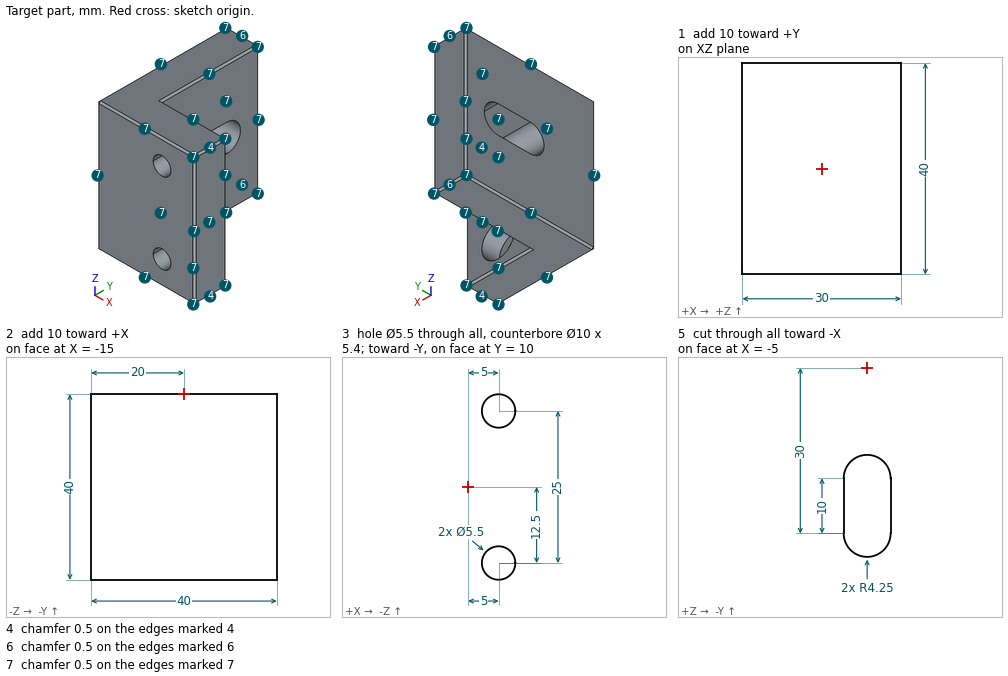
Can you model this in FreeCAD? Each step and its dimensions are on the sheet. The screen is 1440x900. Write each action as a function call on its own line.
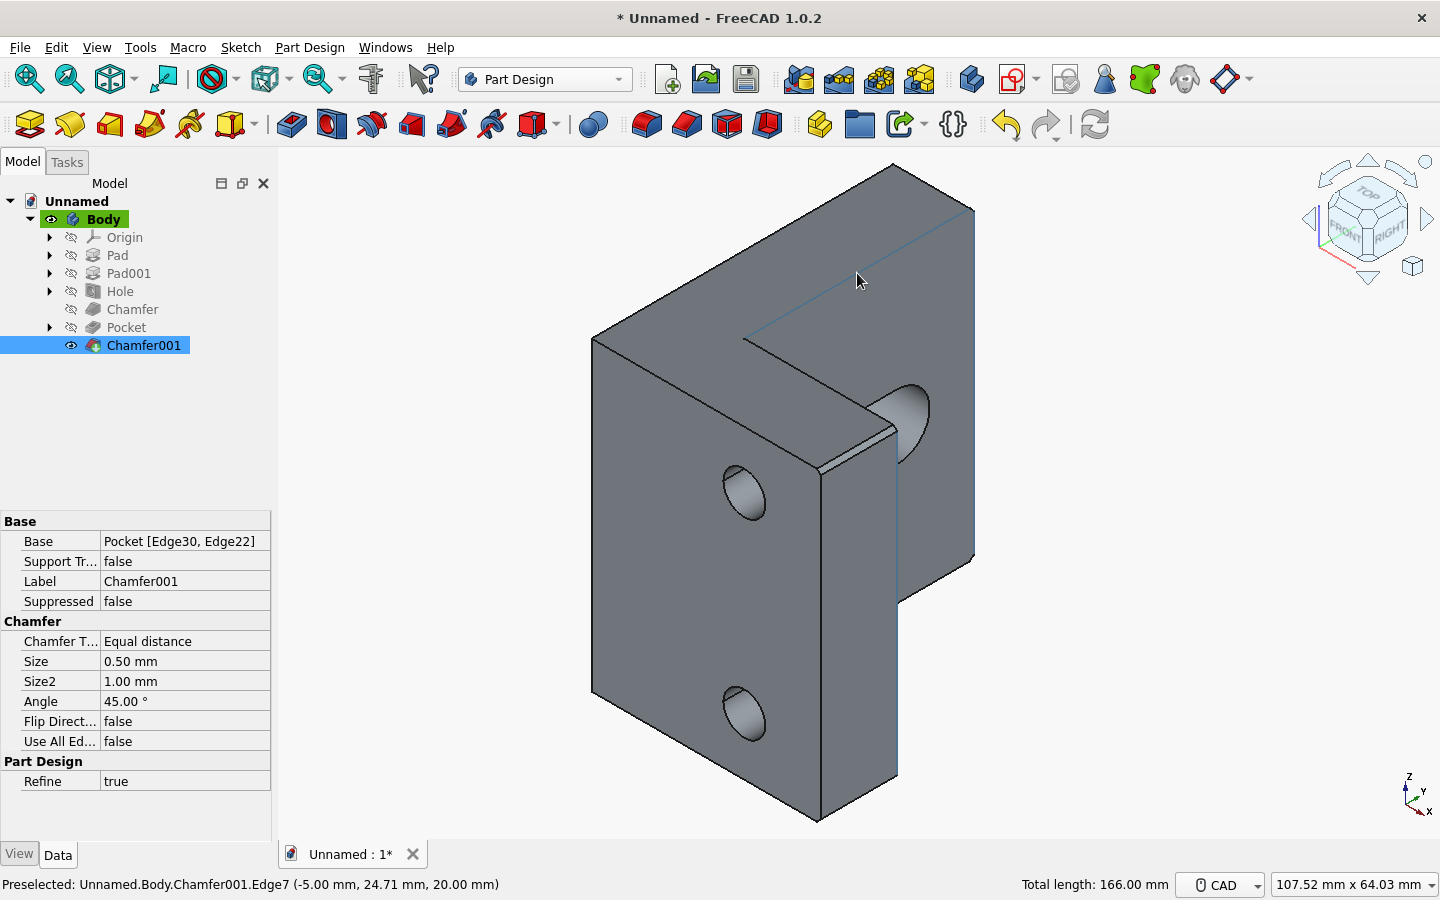
click(704, 403, ctrl)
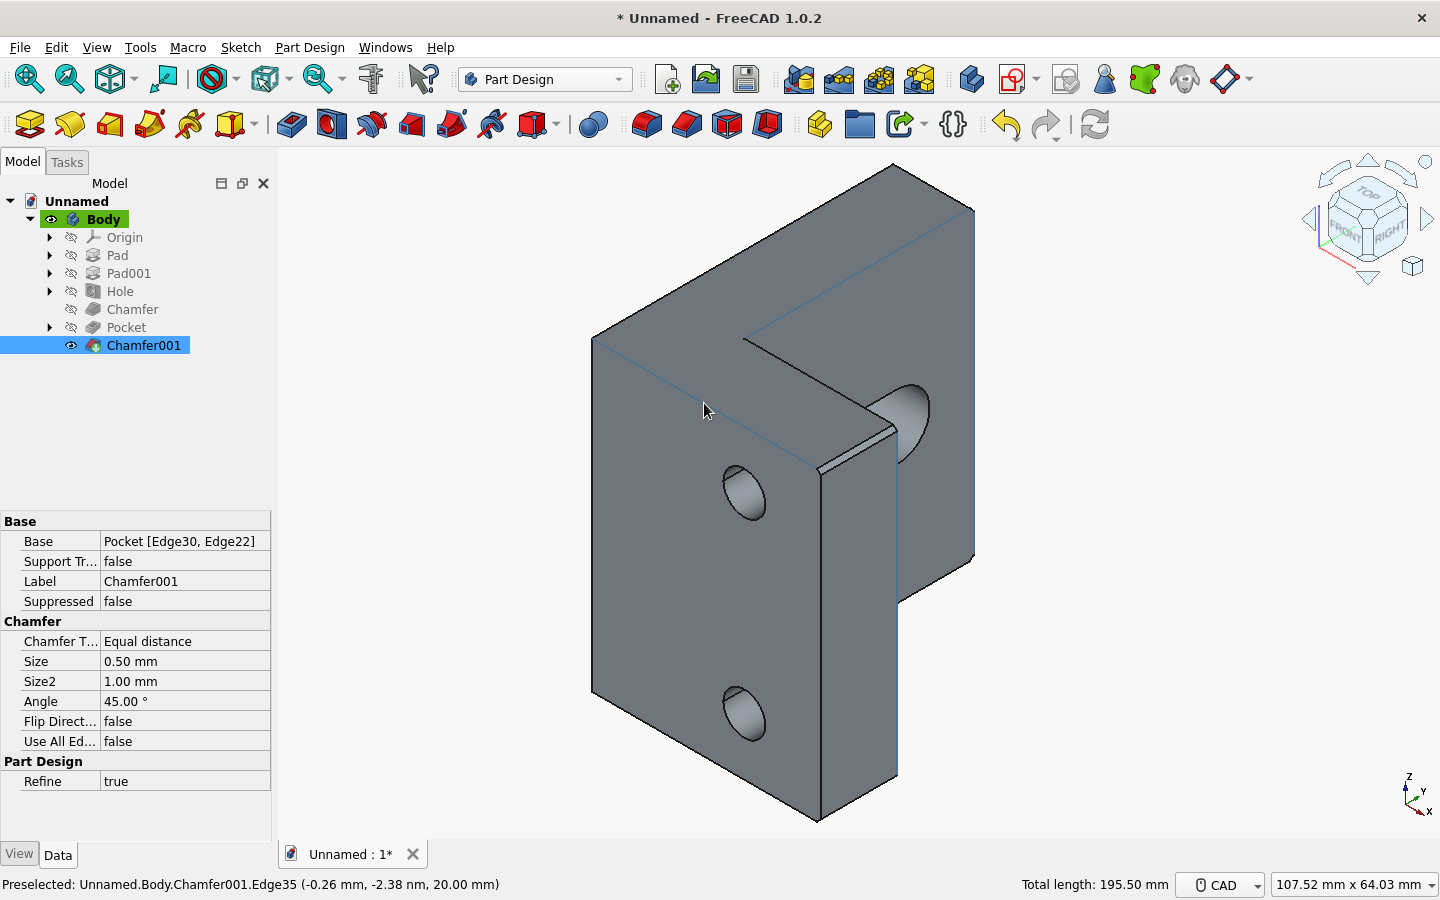
click(821, 646, ctrl)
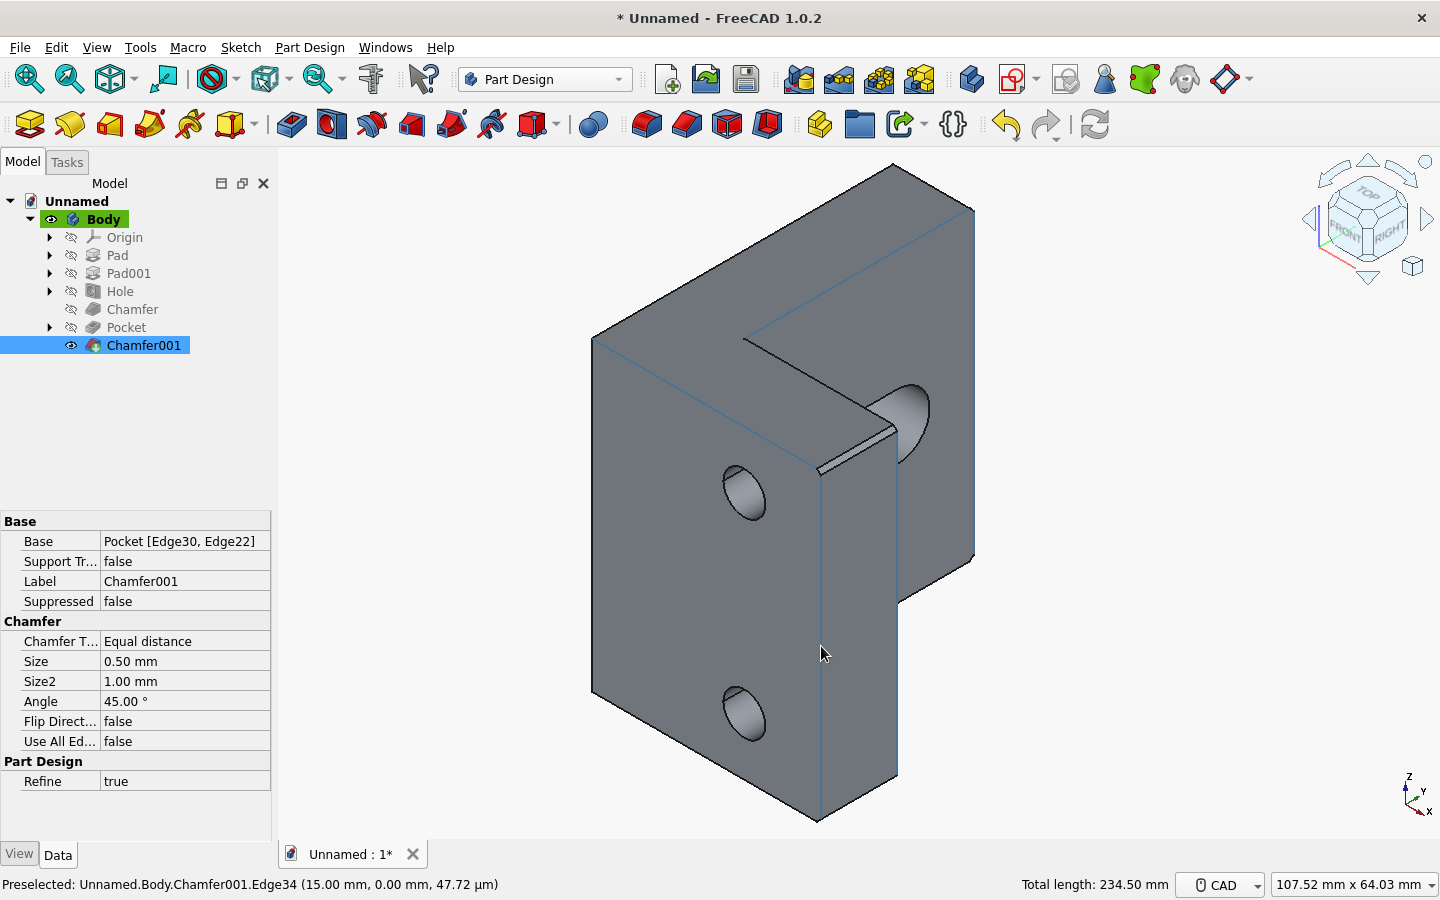
key(2)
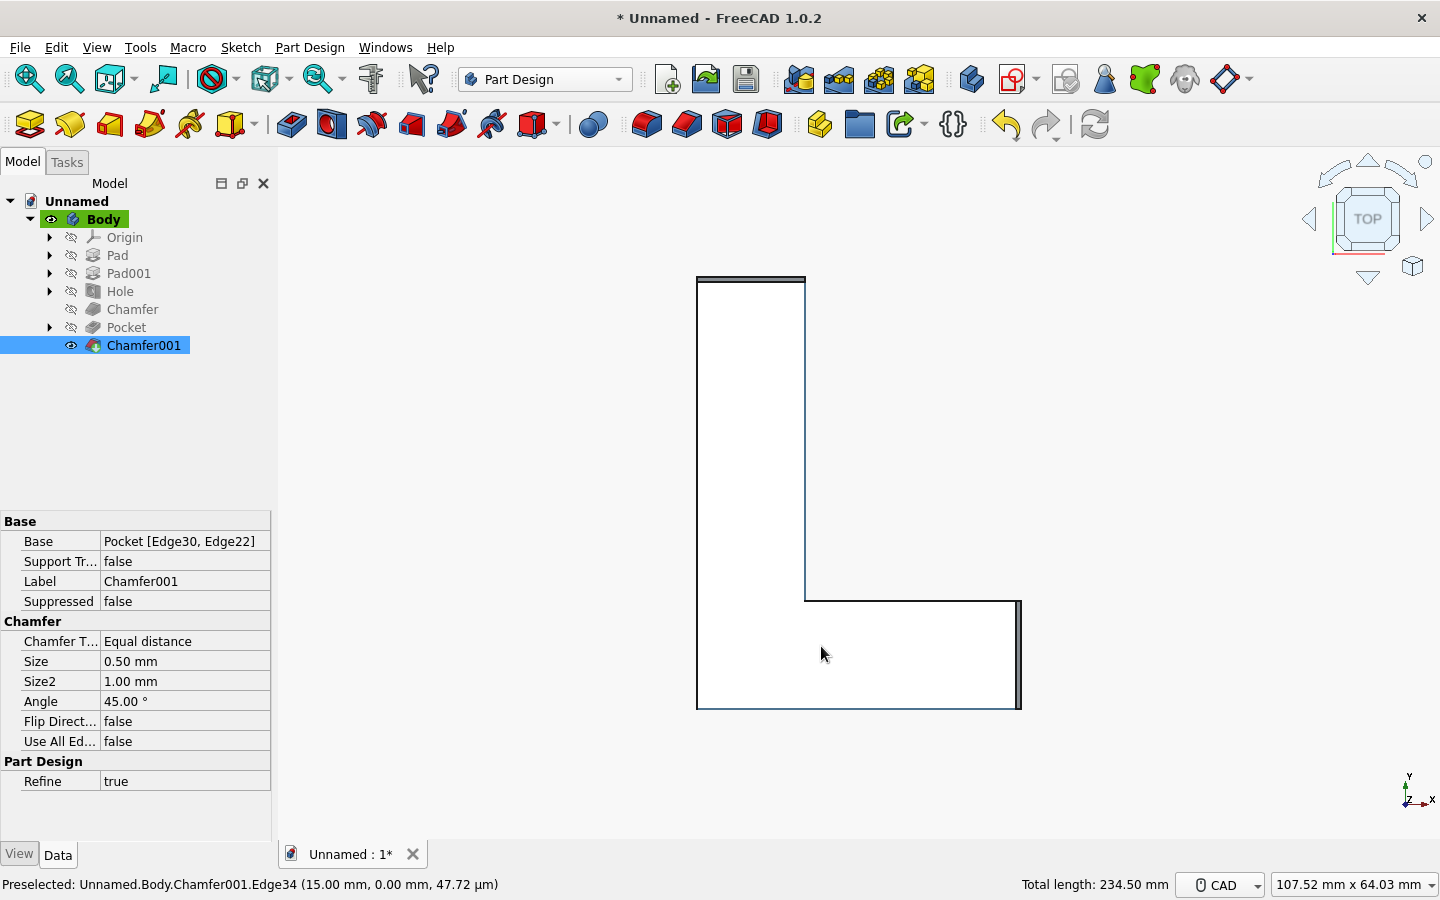
click(910, 600, ctrl)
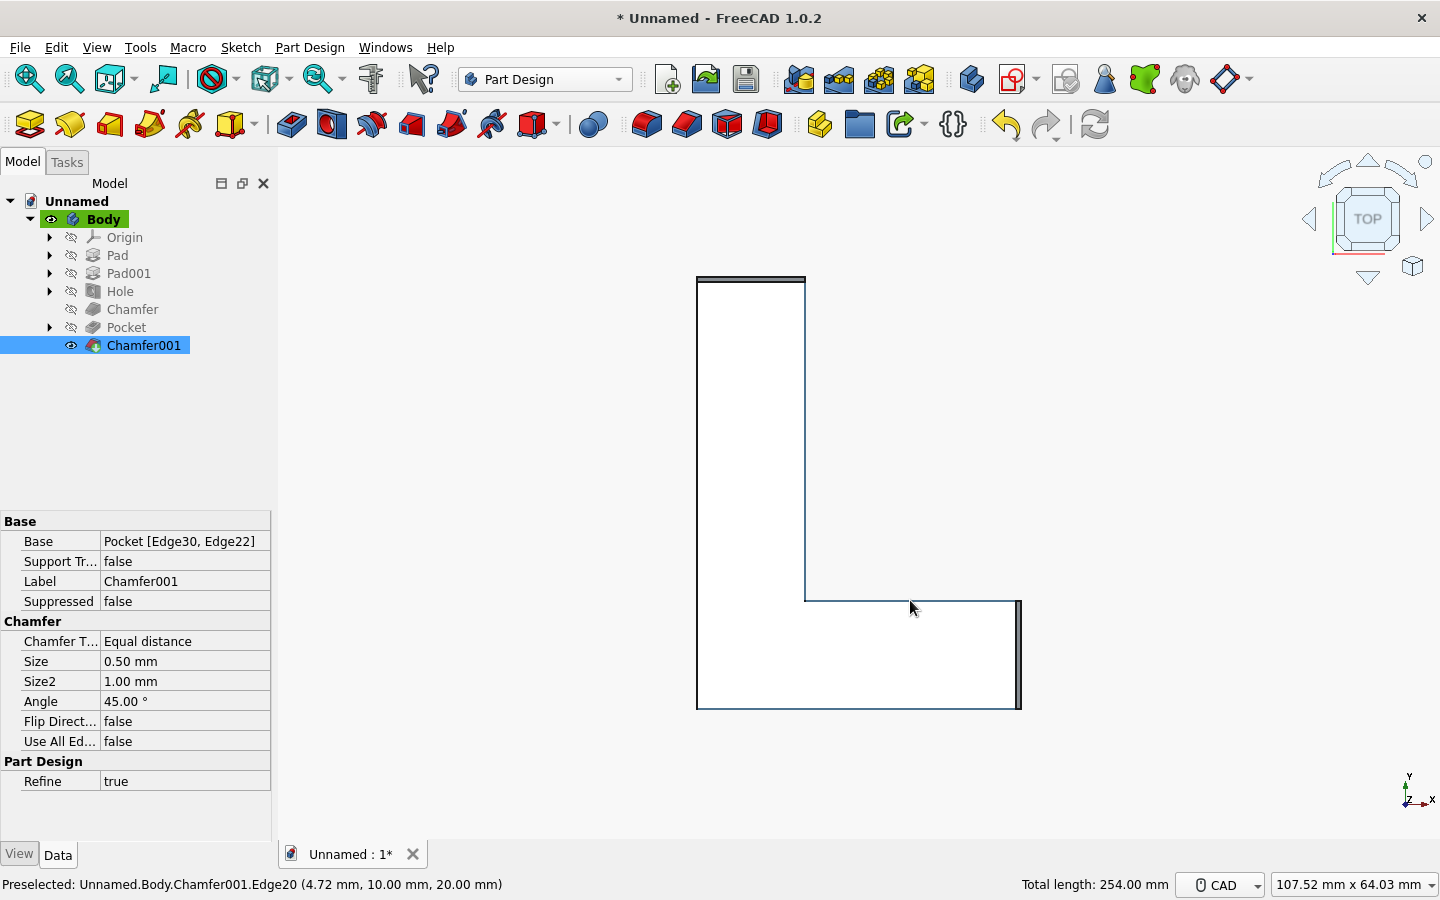
click(697, 495, ctrl)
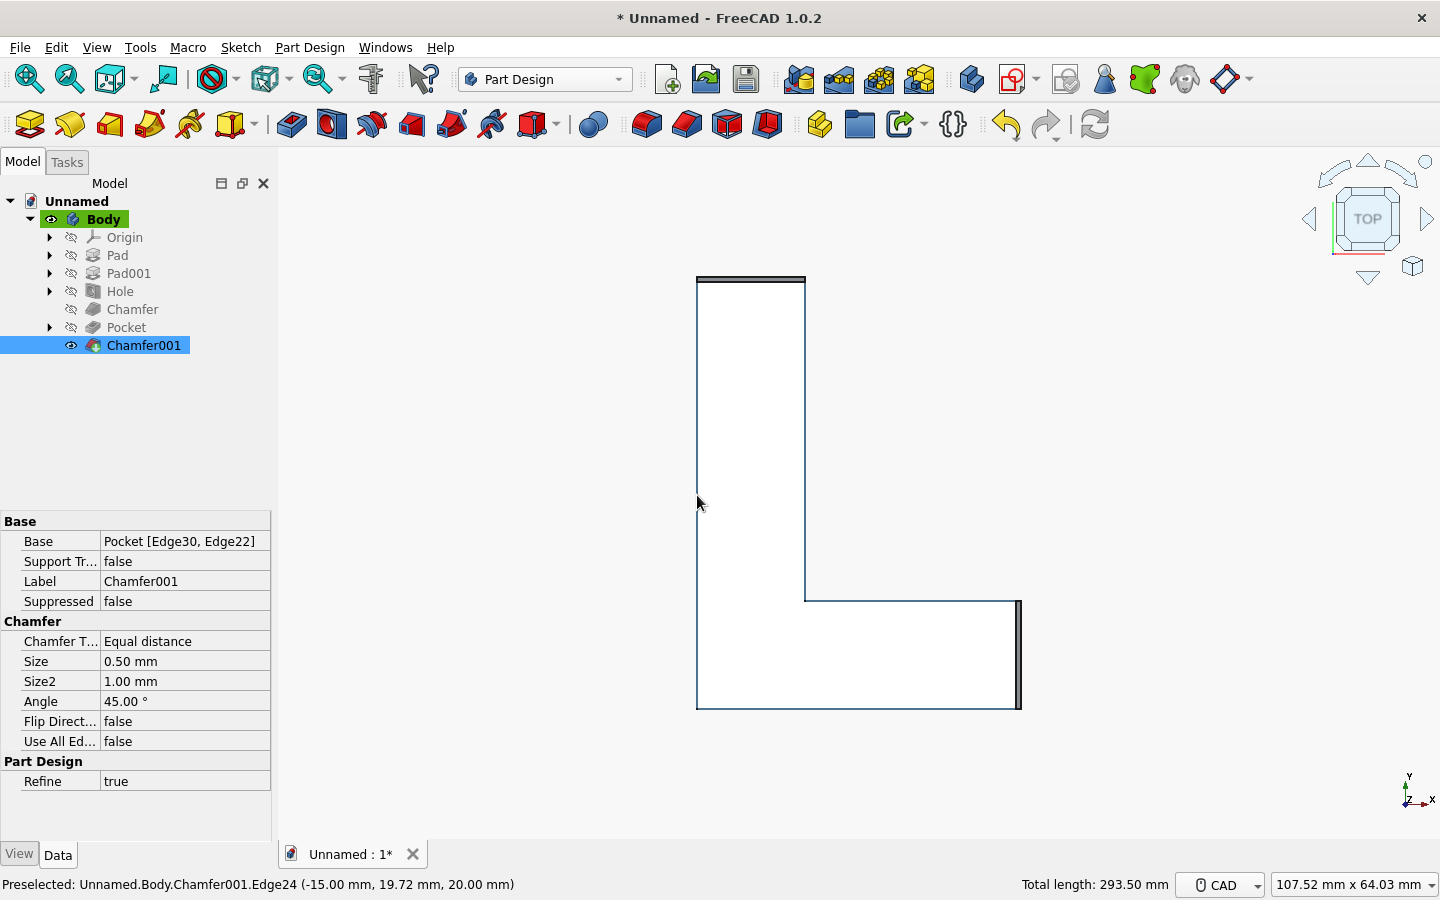
key(1)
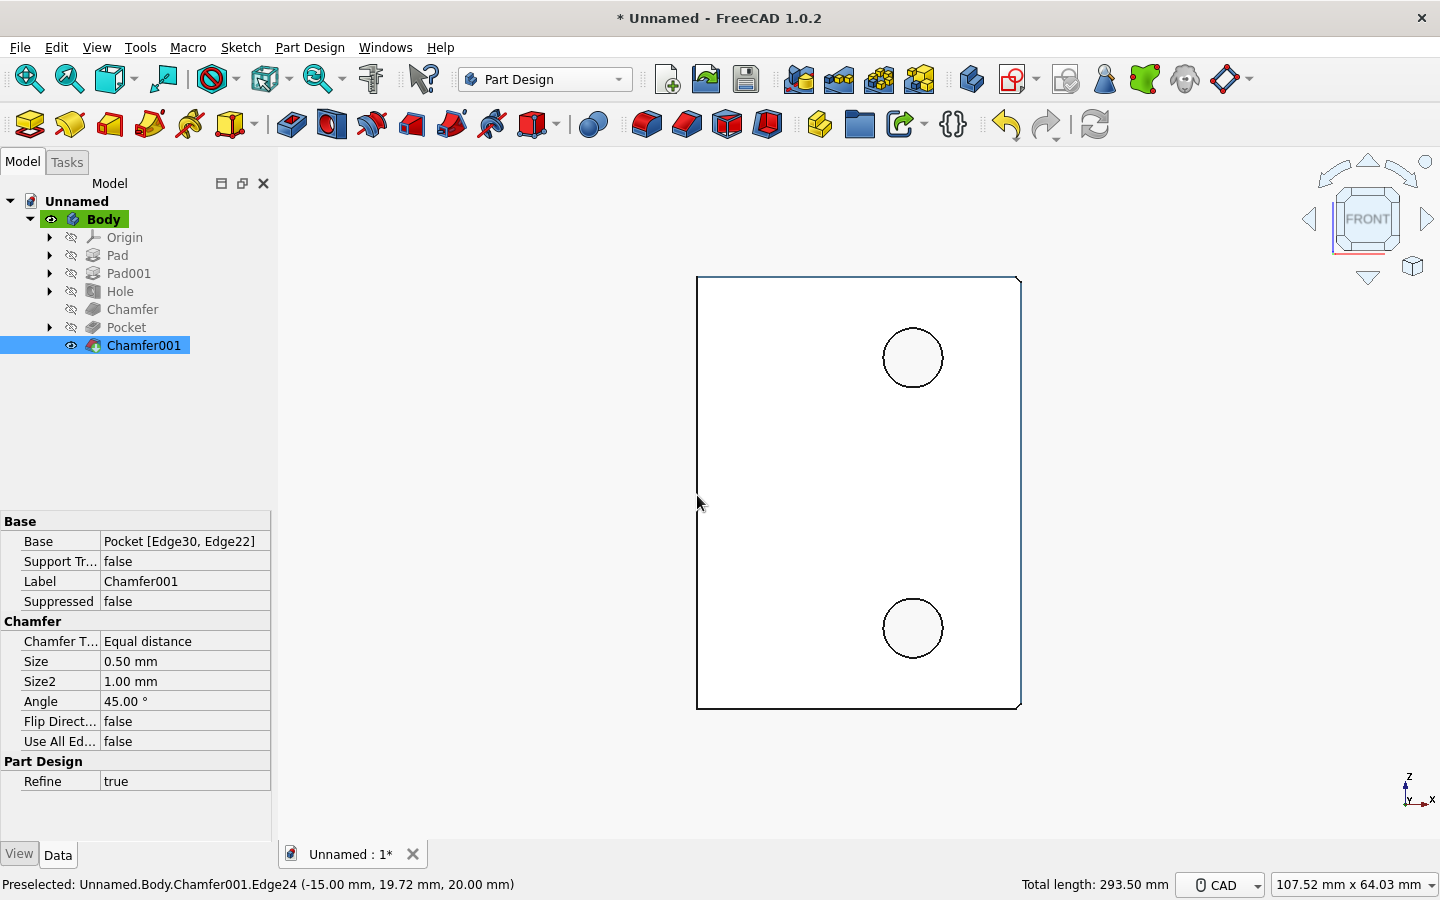
click(697, 492, ctrl)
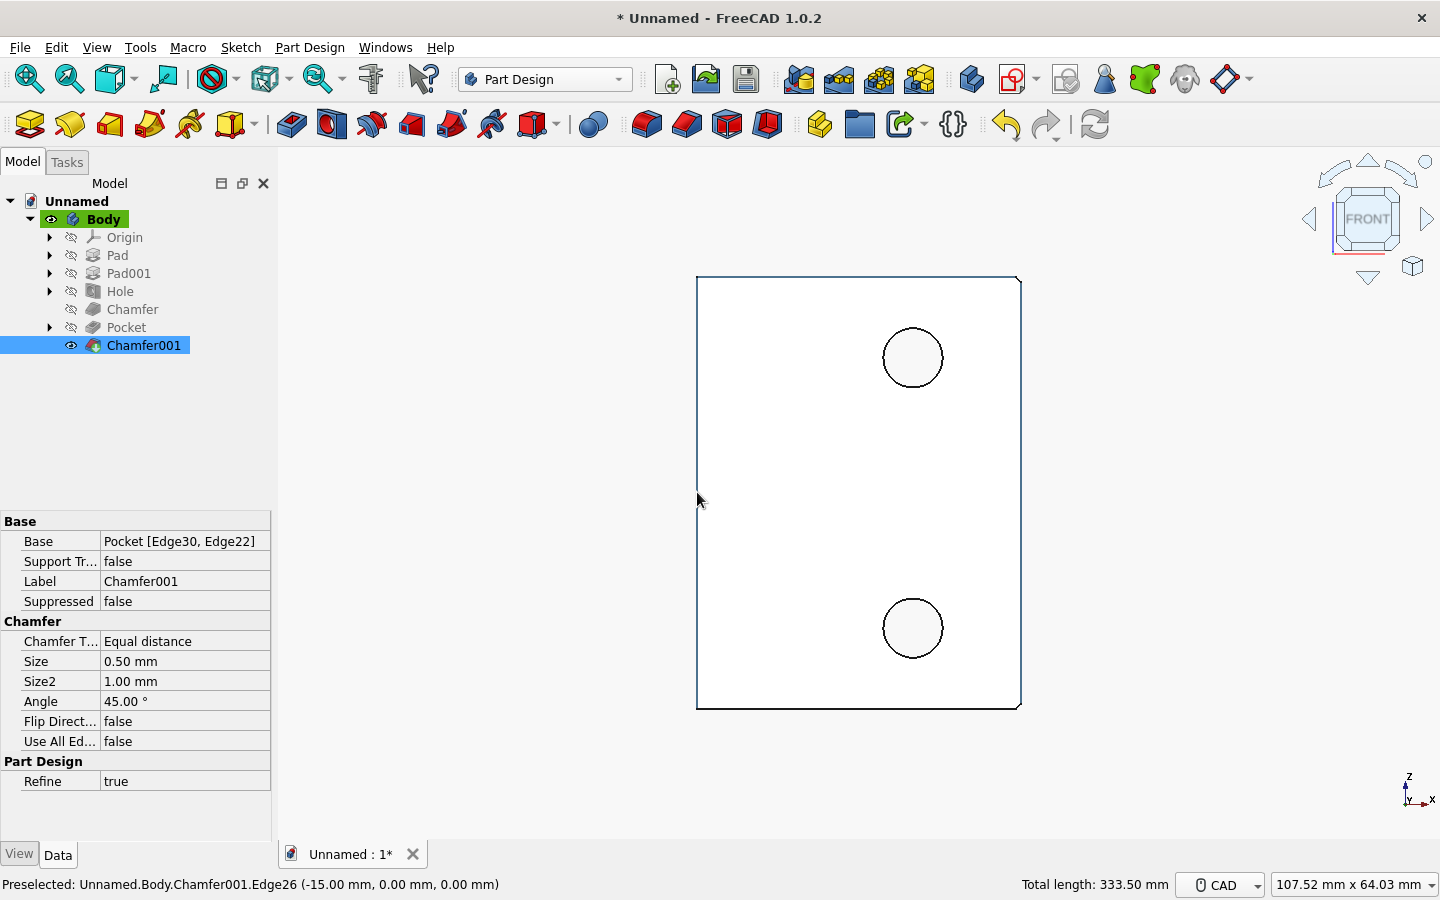
key(3)